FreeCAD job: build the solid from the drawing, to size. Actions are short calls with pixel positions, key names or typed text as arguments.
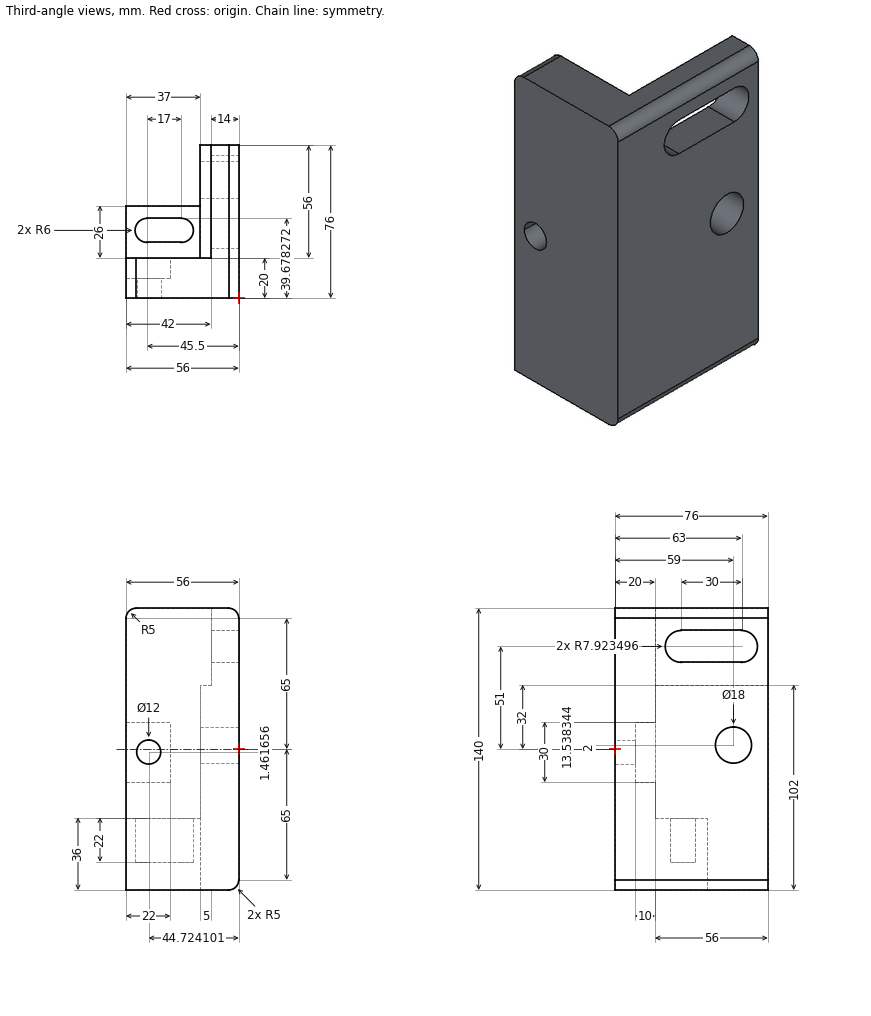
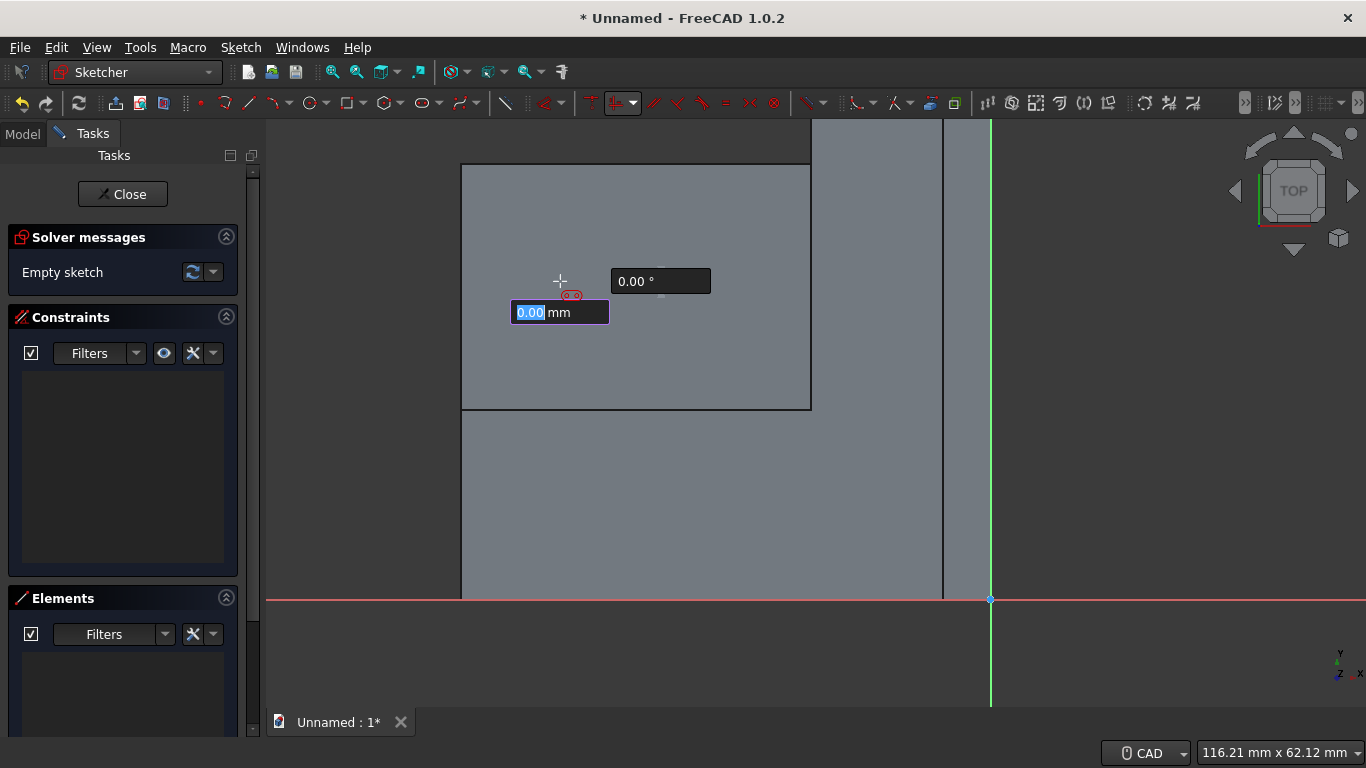
click(721, 281)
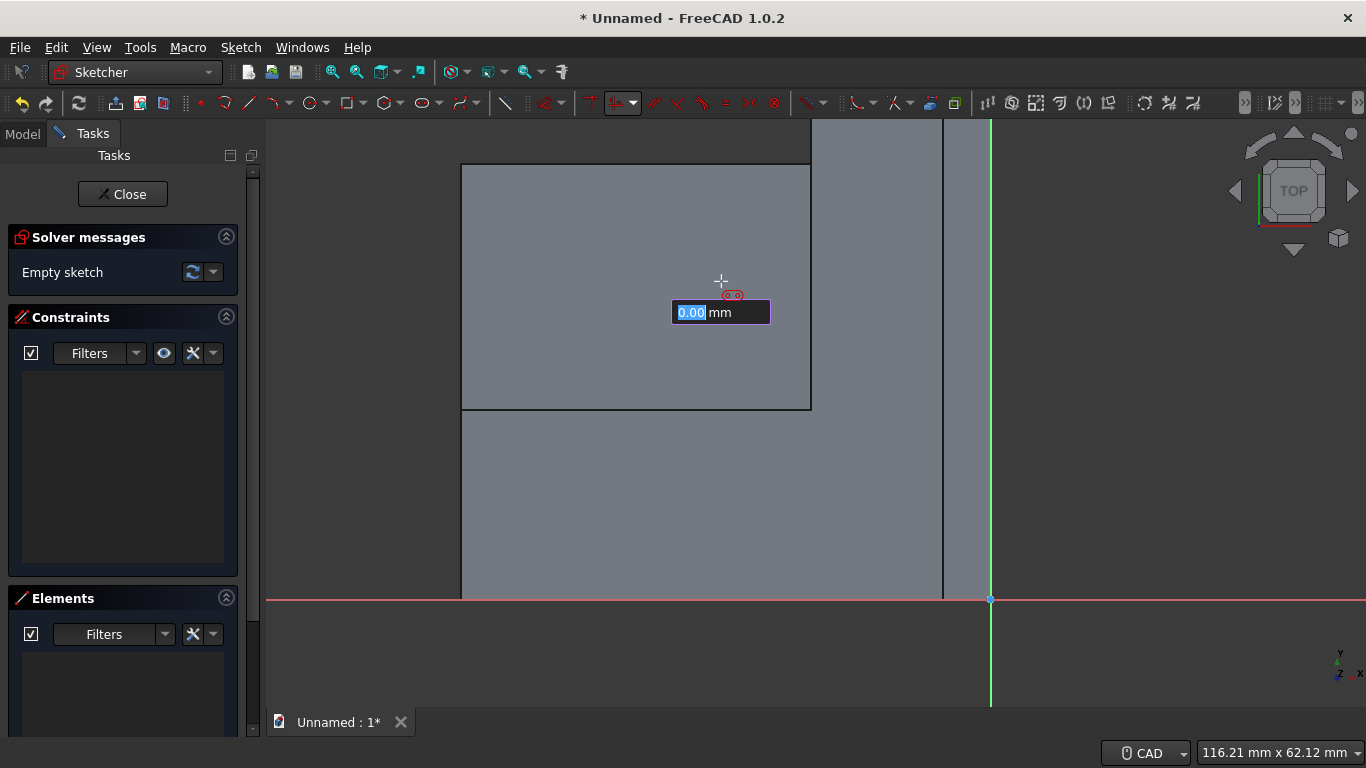
click(641, 224)
key(Escape)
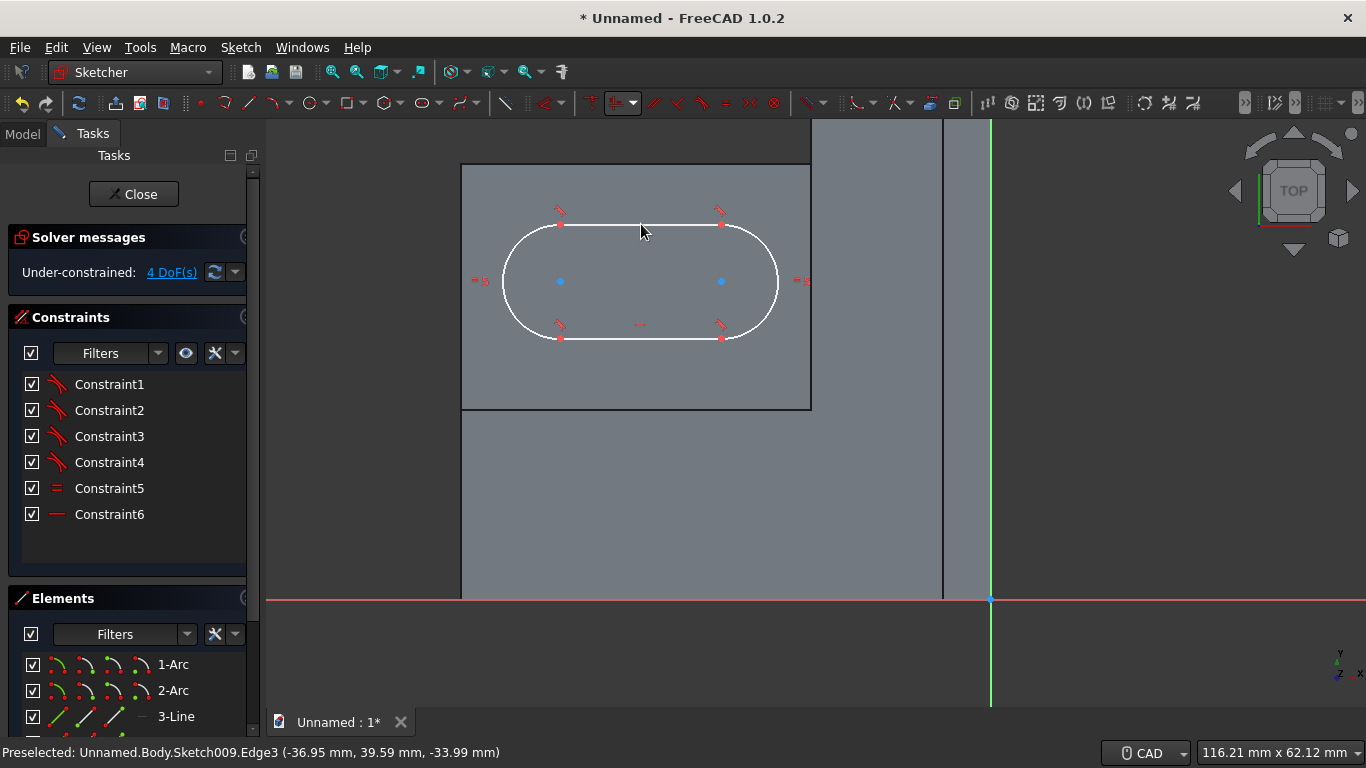
key(d)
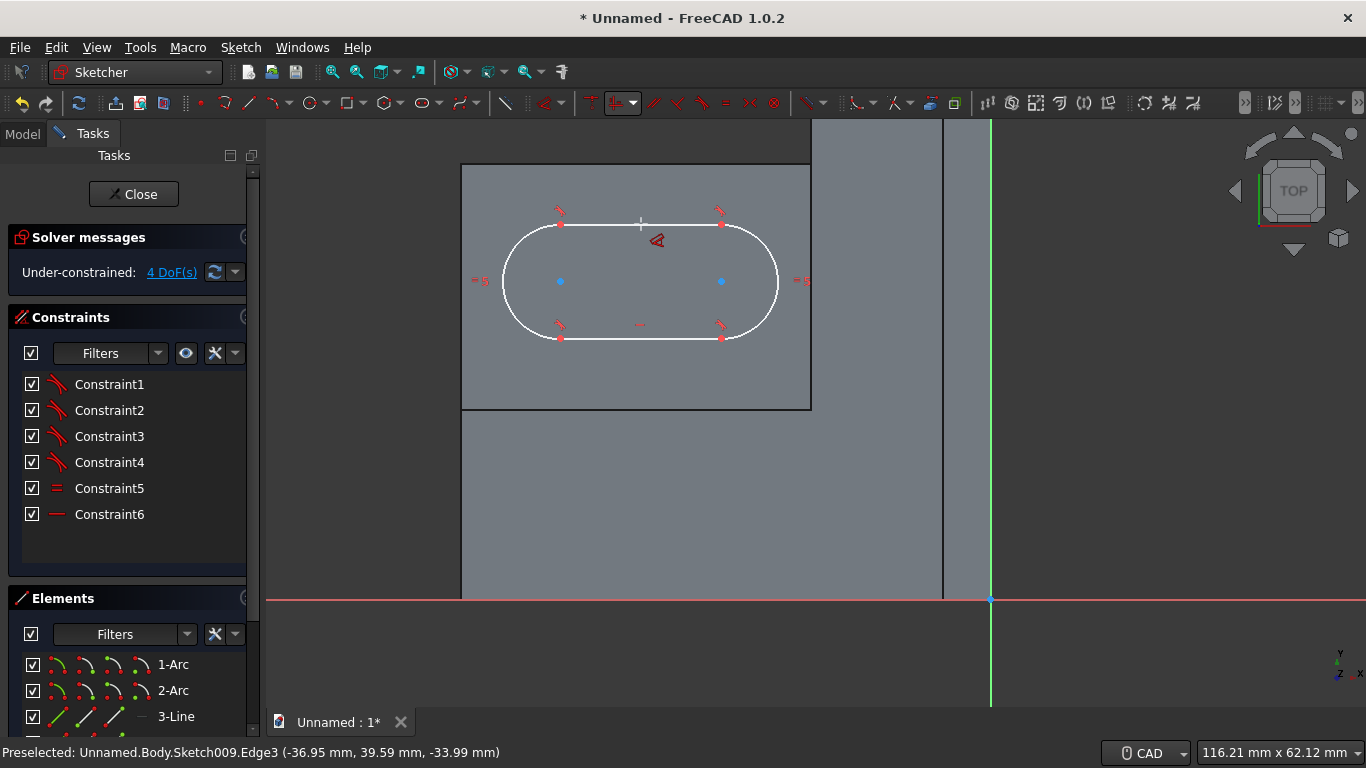
click(514, 248)
click(488, 229)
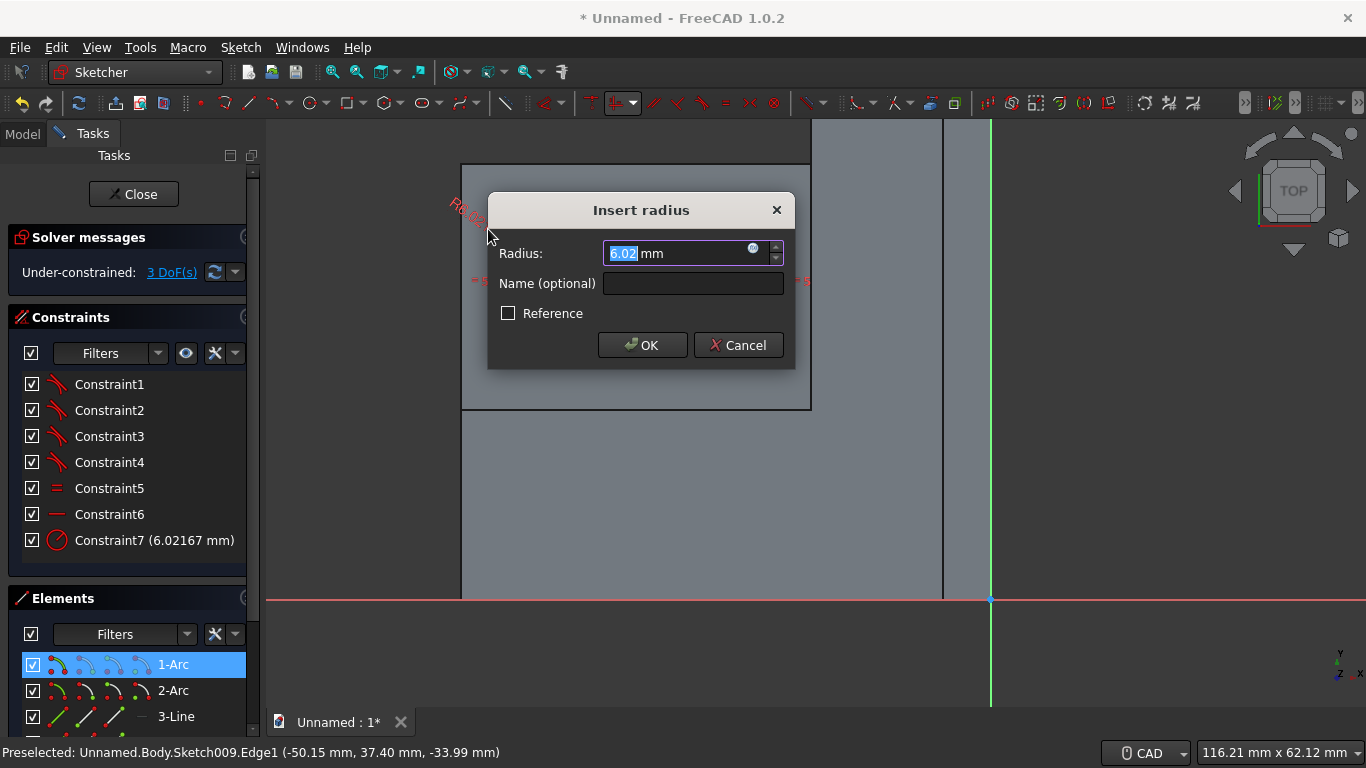
text(6)
key(Return)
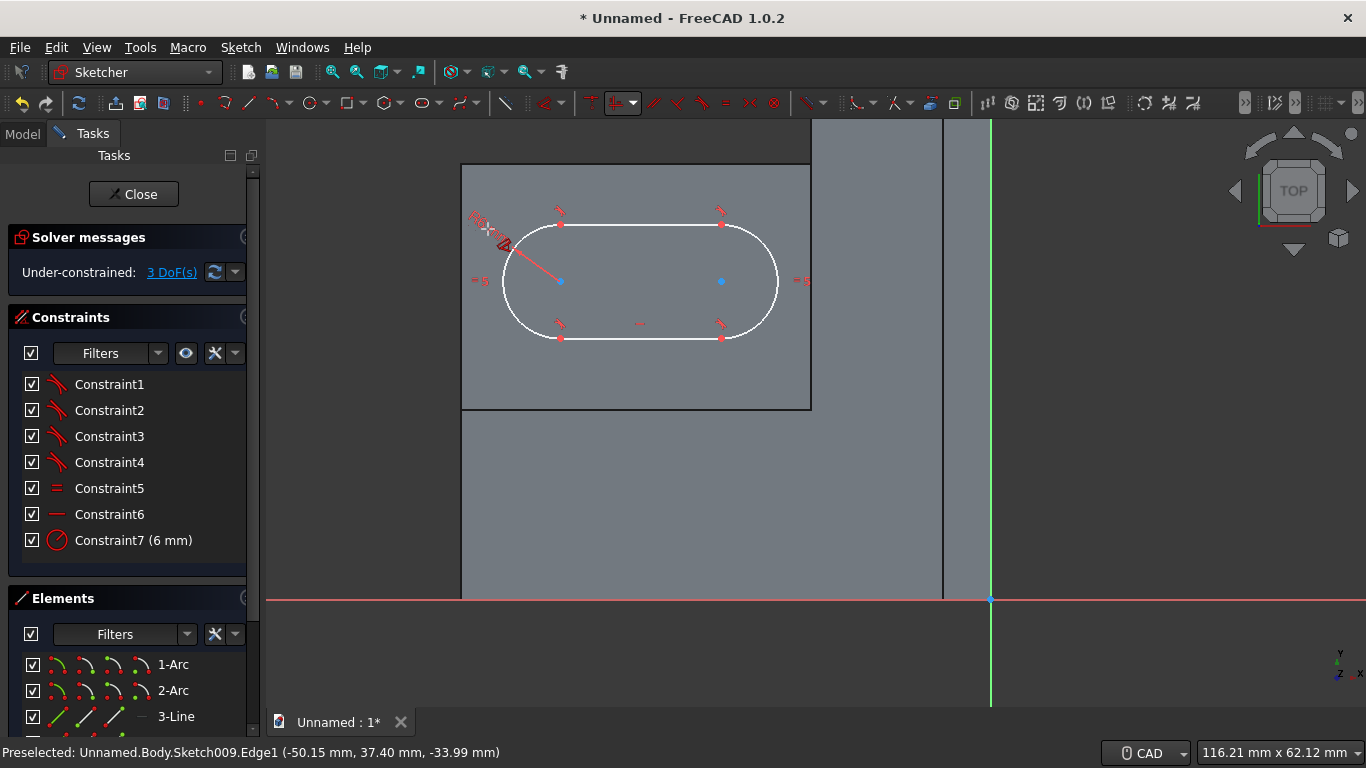
click(608, 225)
click(641, 191)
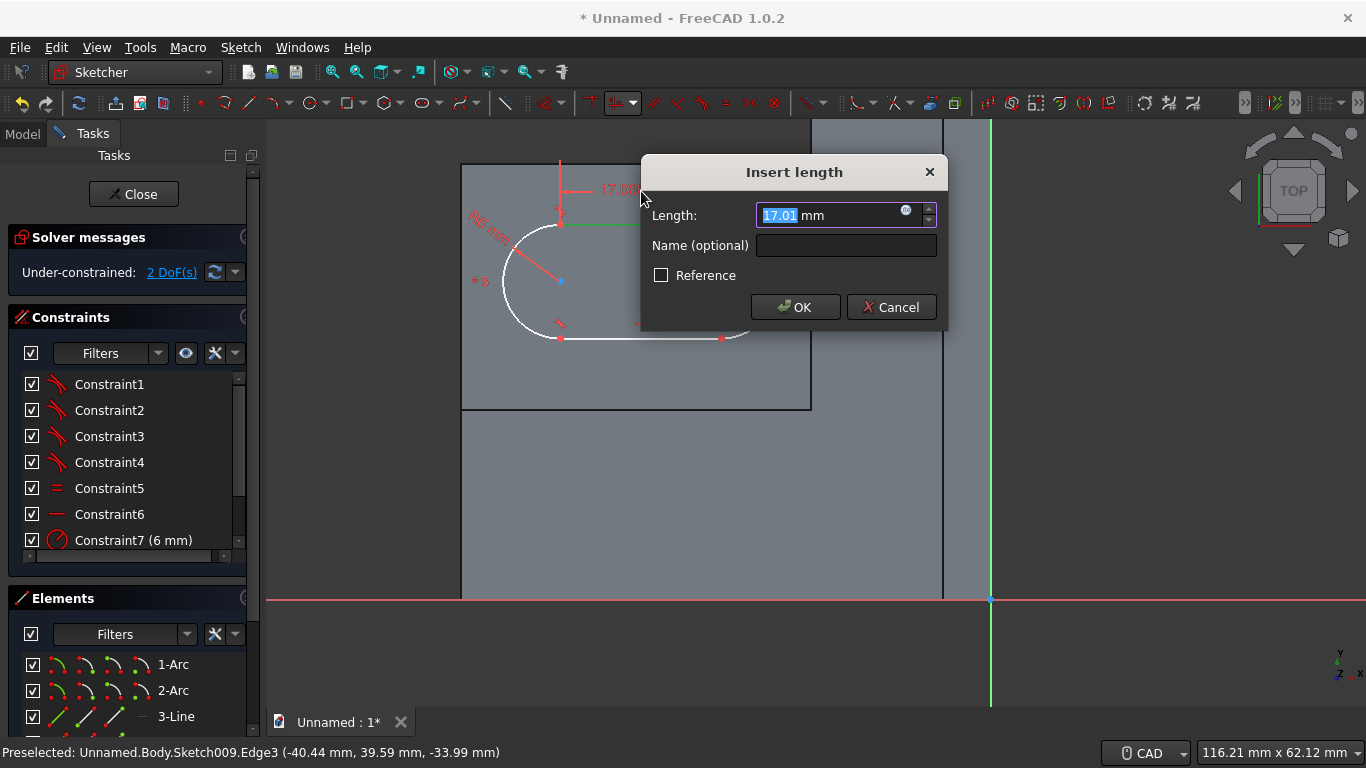
text(17)
key(Return)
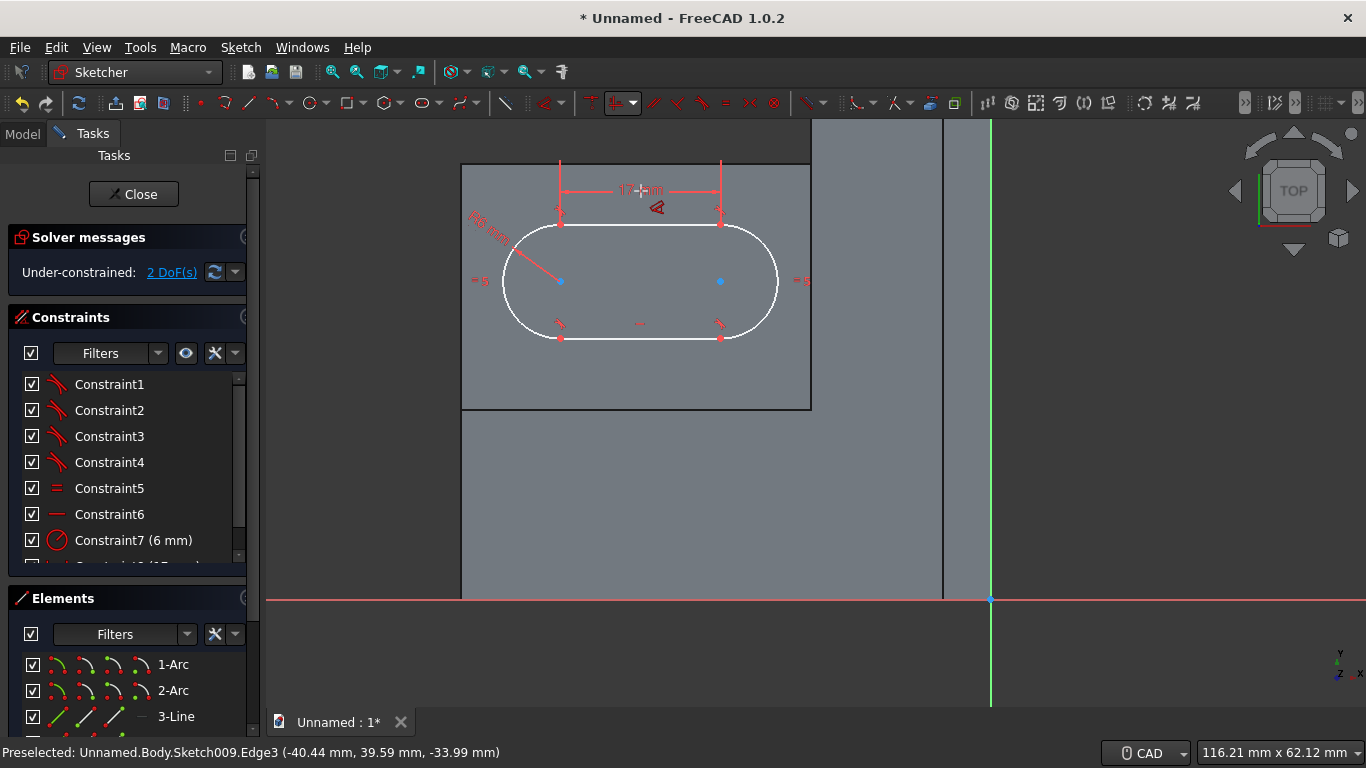
click(560, 225)
click(775, 634)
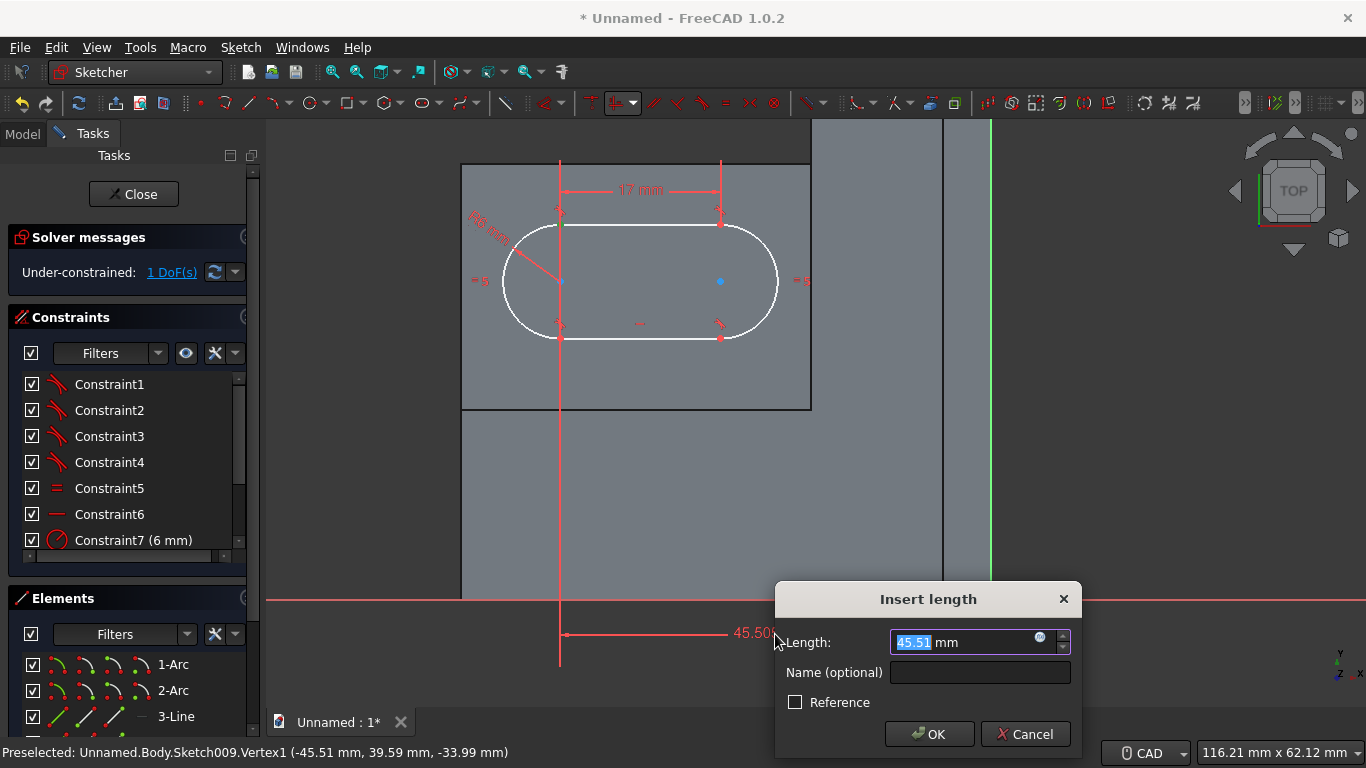
text(45.5)
key(Return)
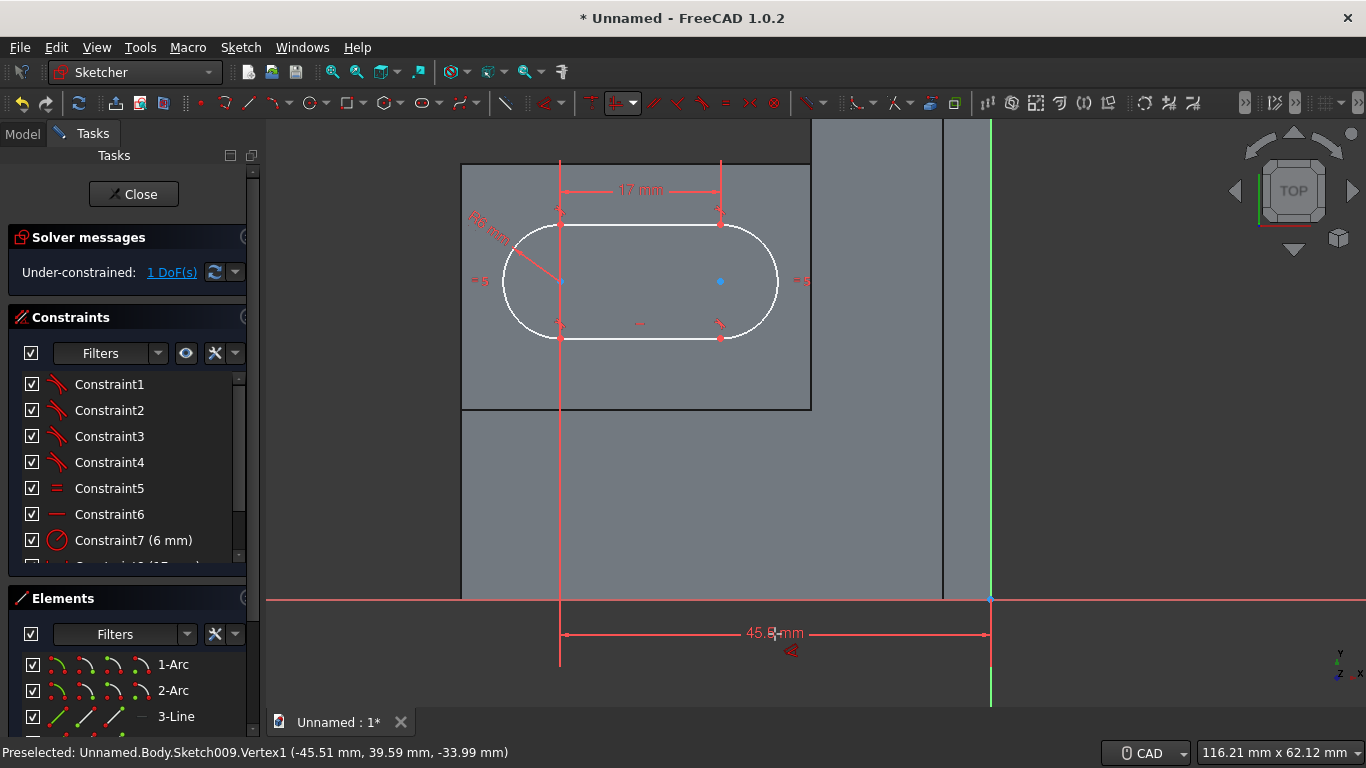
click(560, 225)
click(1025, 412)